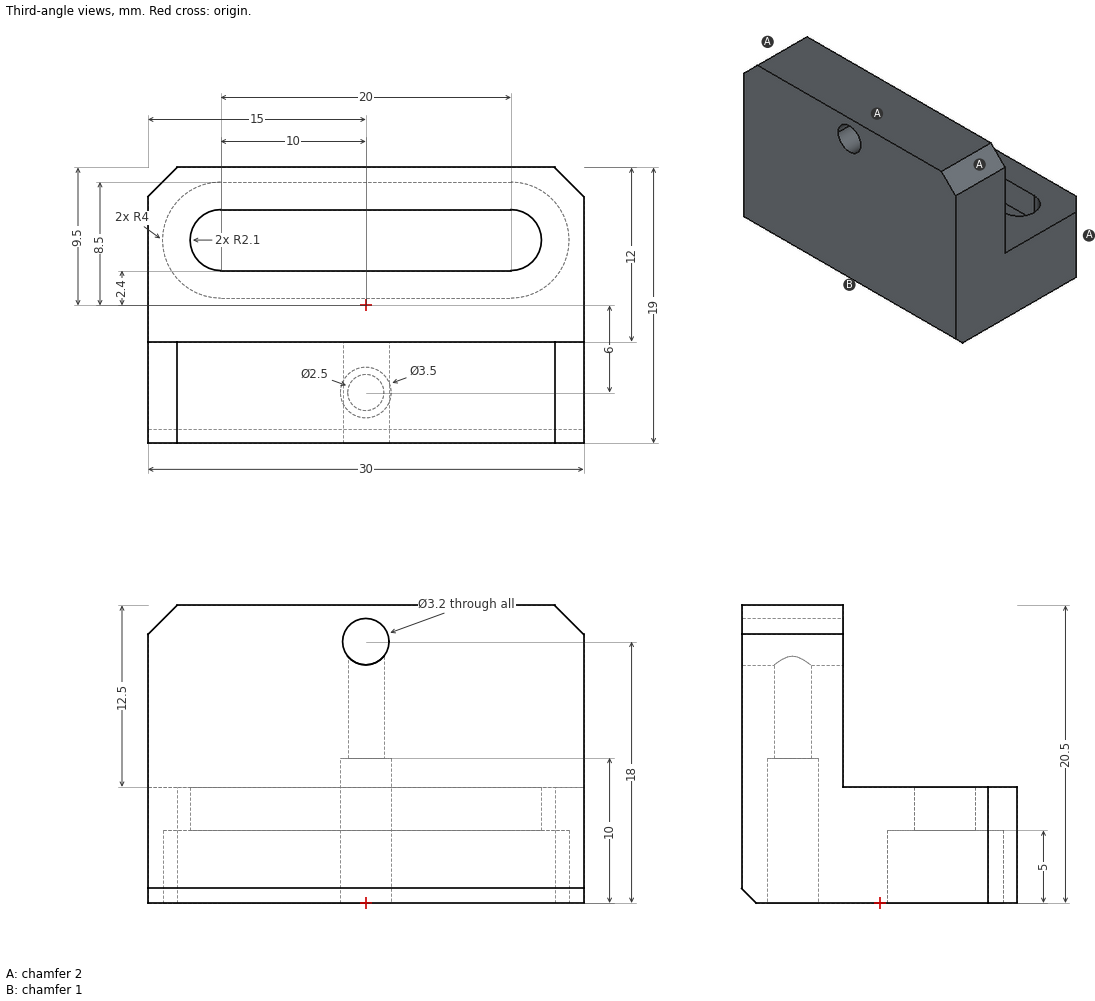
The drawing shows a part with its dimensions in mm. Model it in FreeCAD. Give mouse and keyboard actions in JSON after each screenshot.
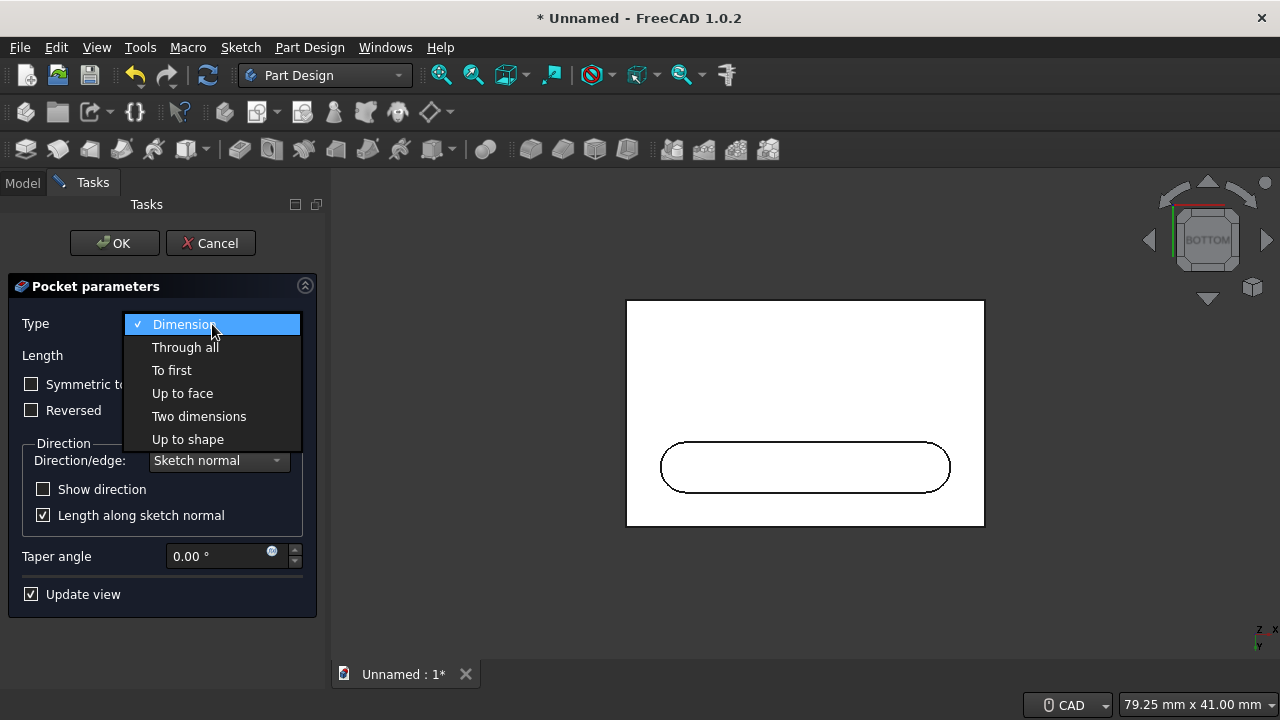
{"action": "left_click", "coordinate": [212, 348]}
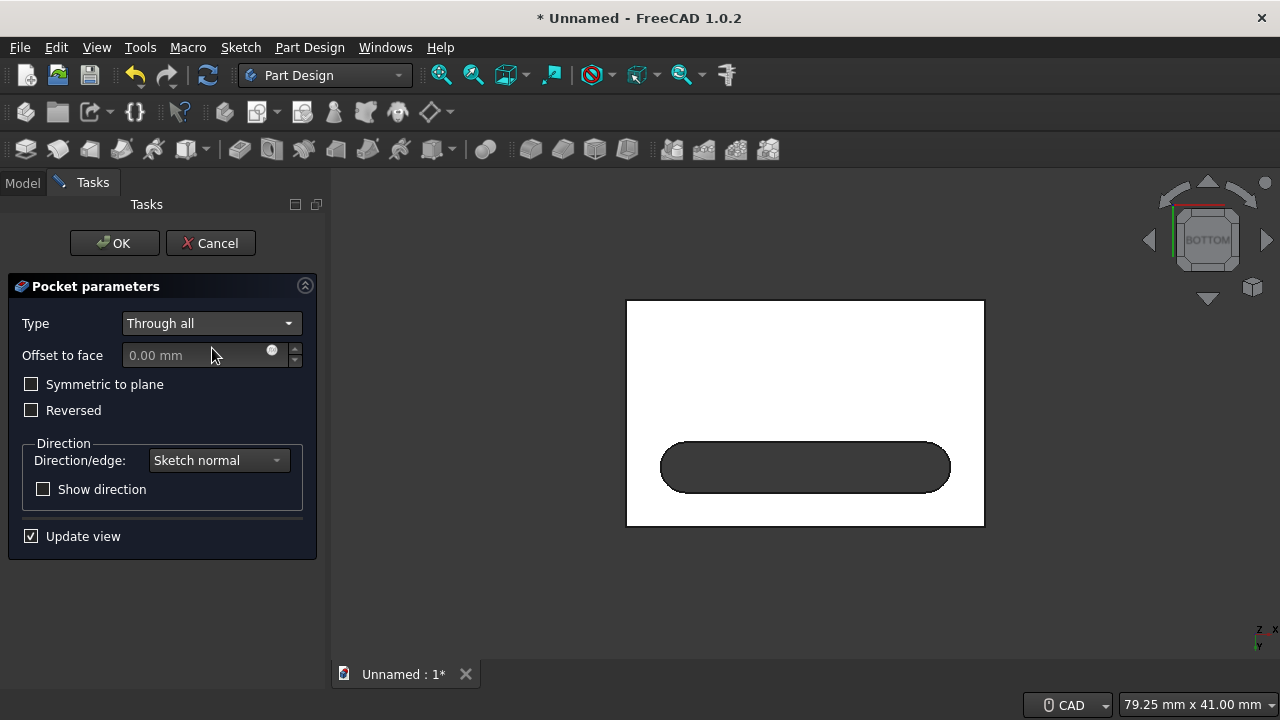
{"action": "left_click", "coordinate": [115, 243]}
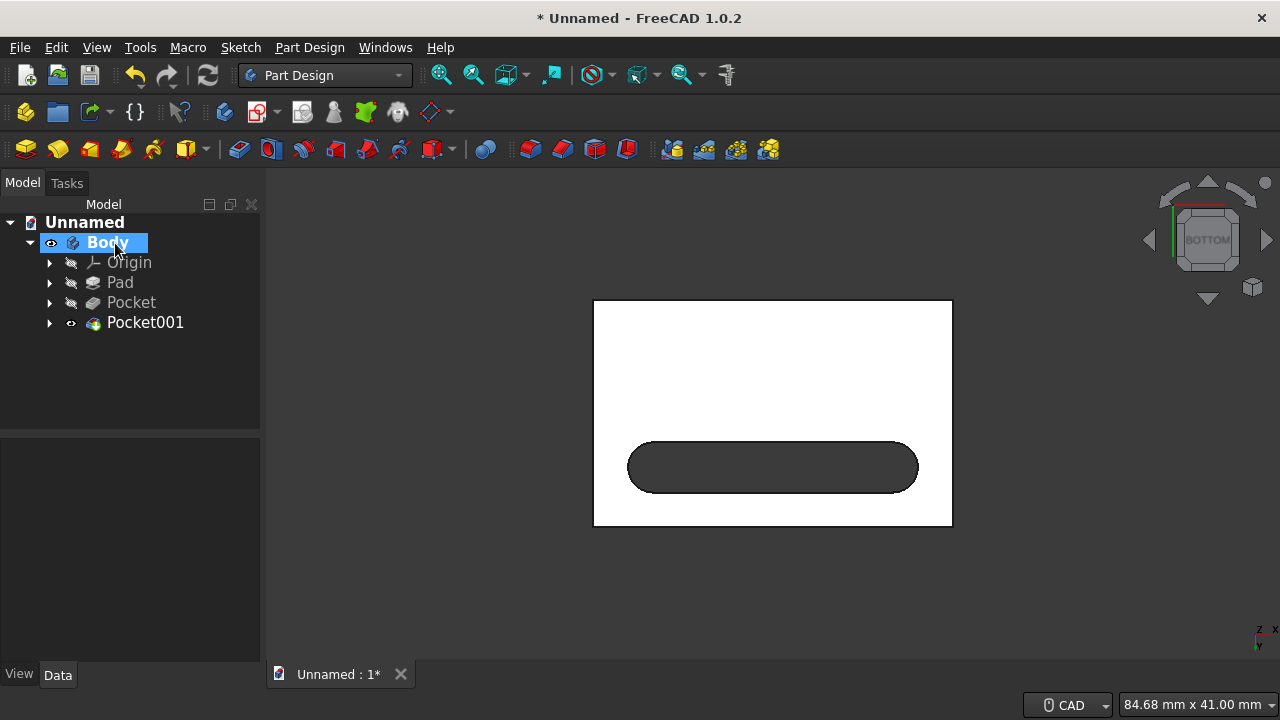
{"action": "left_click", "coordinate": [258, 112]}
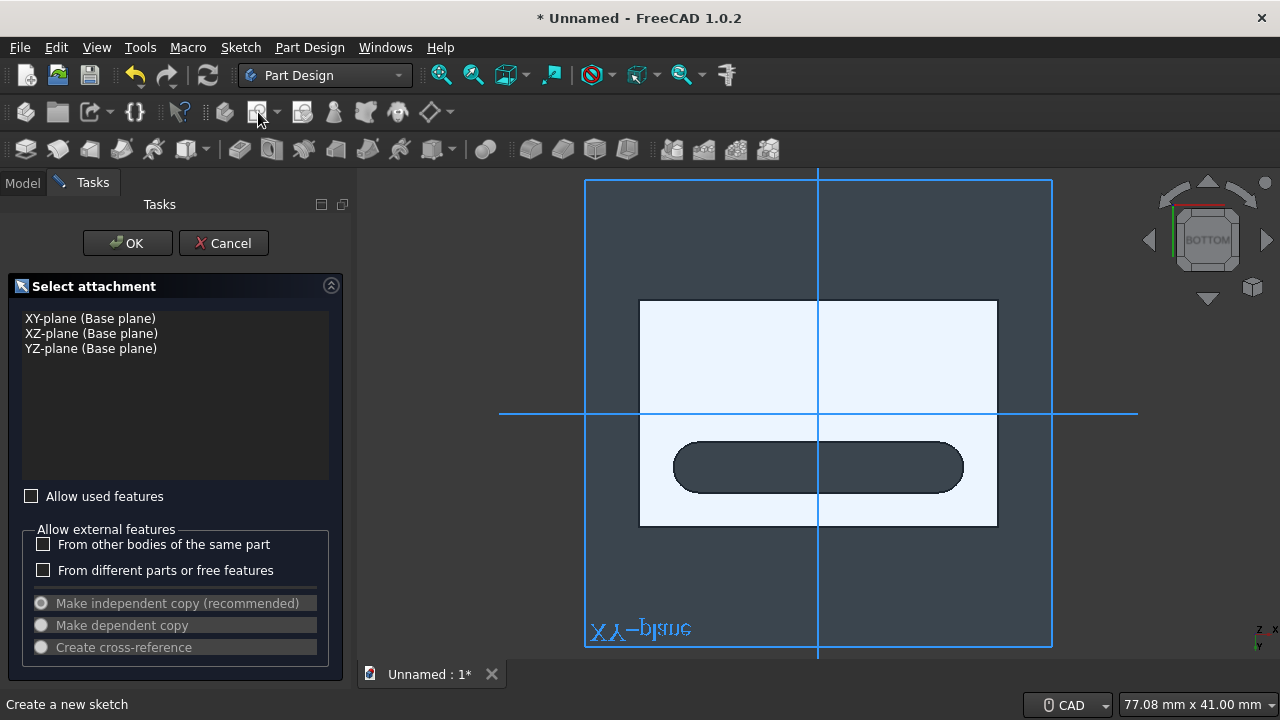
{"action": "left_click", "coordinate": [82, 318]}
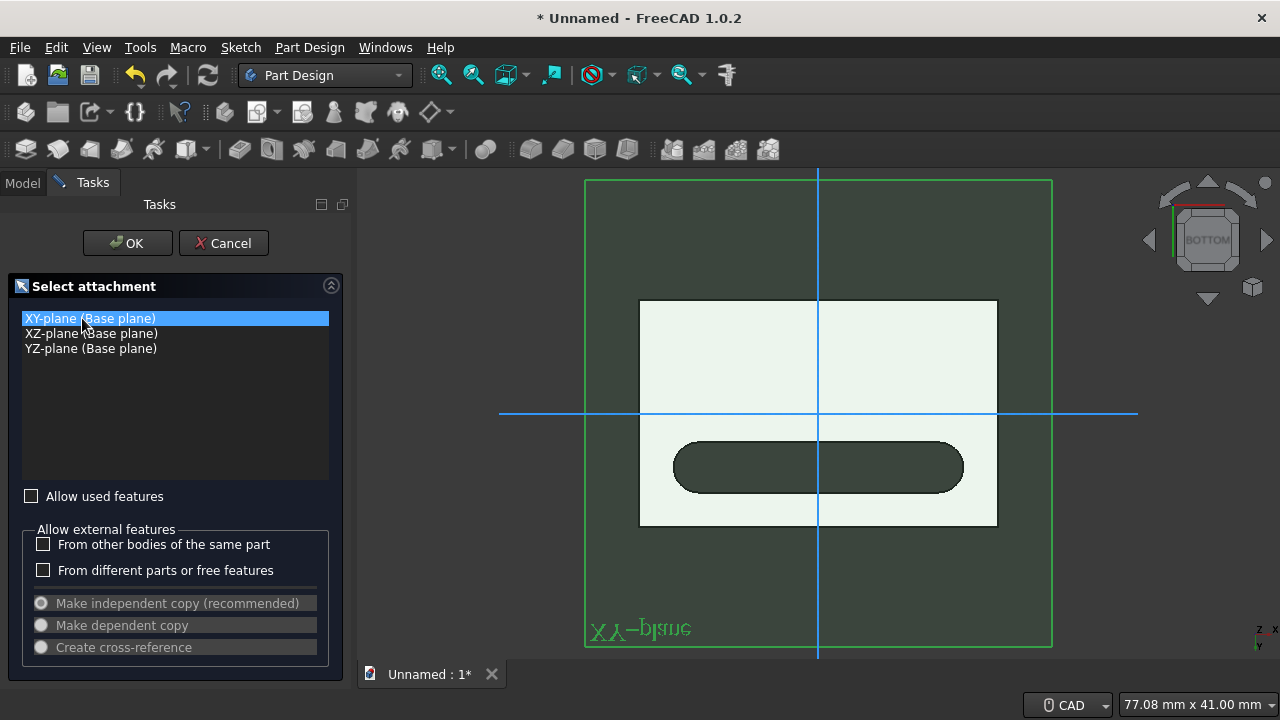
{"action": "left_click", "coordinate": [128, 243]}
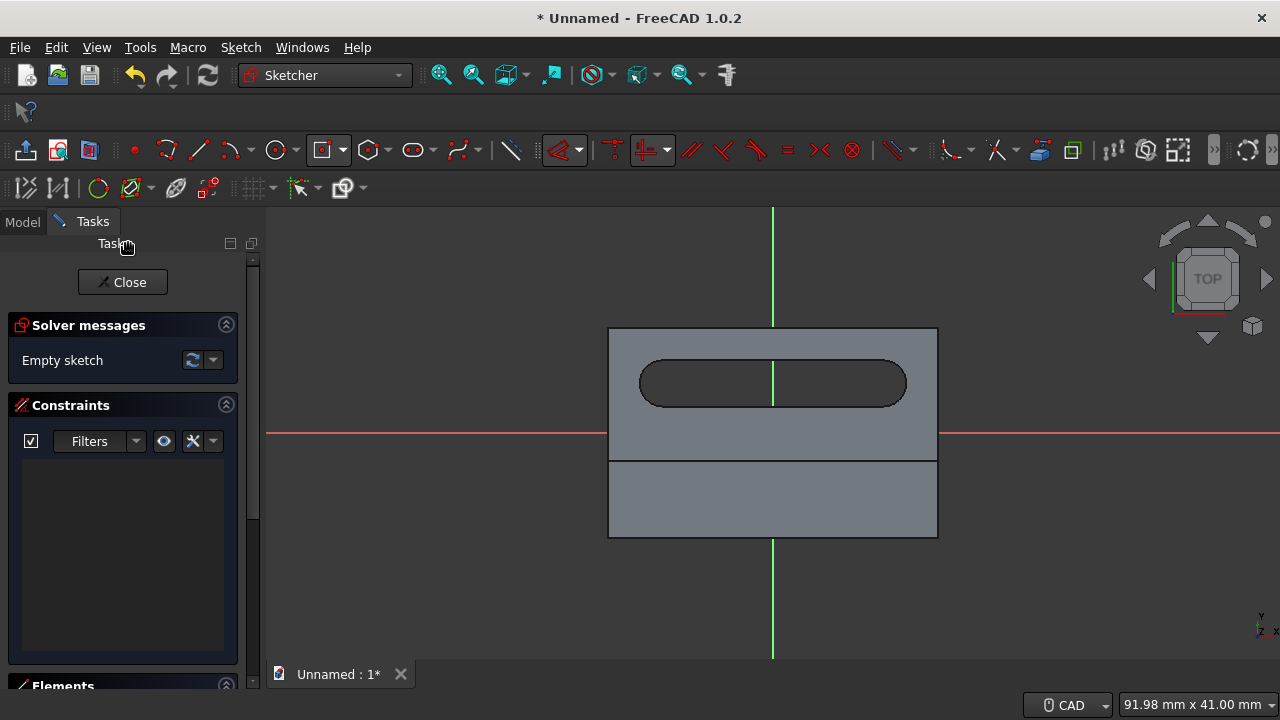
{"action": "left_click", "coordinate": [90, 150]}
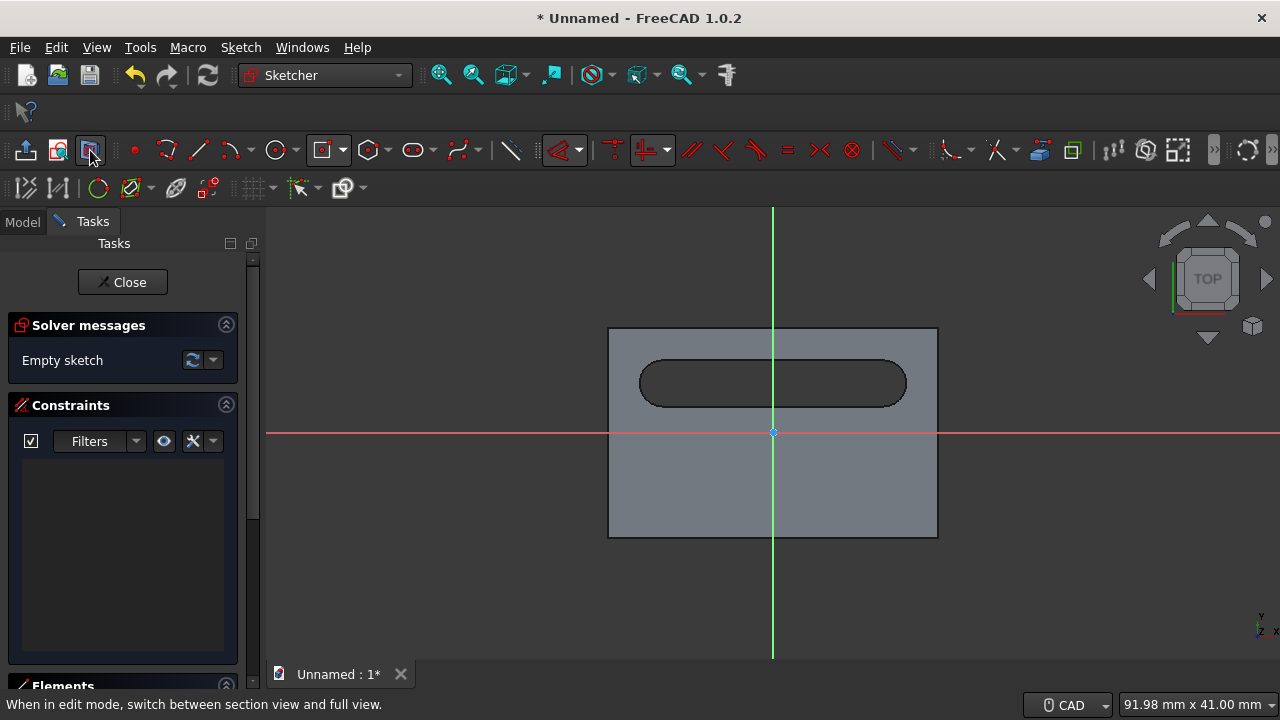
{"action": "scroll", "coordinate": [856, 329], "scroll_direction": "up", "scroll_amount": 3}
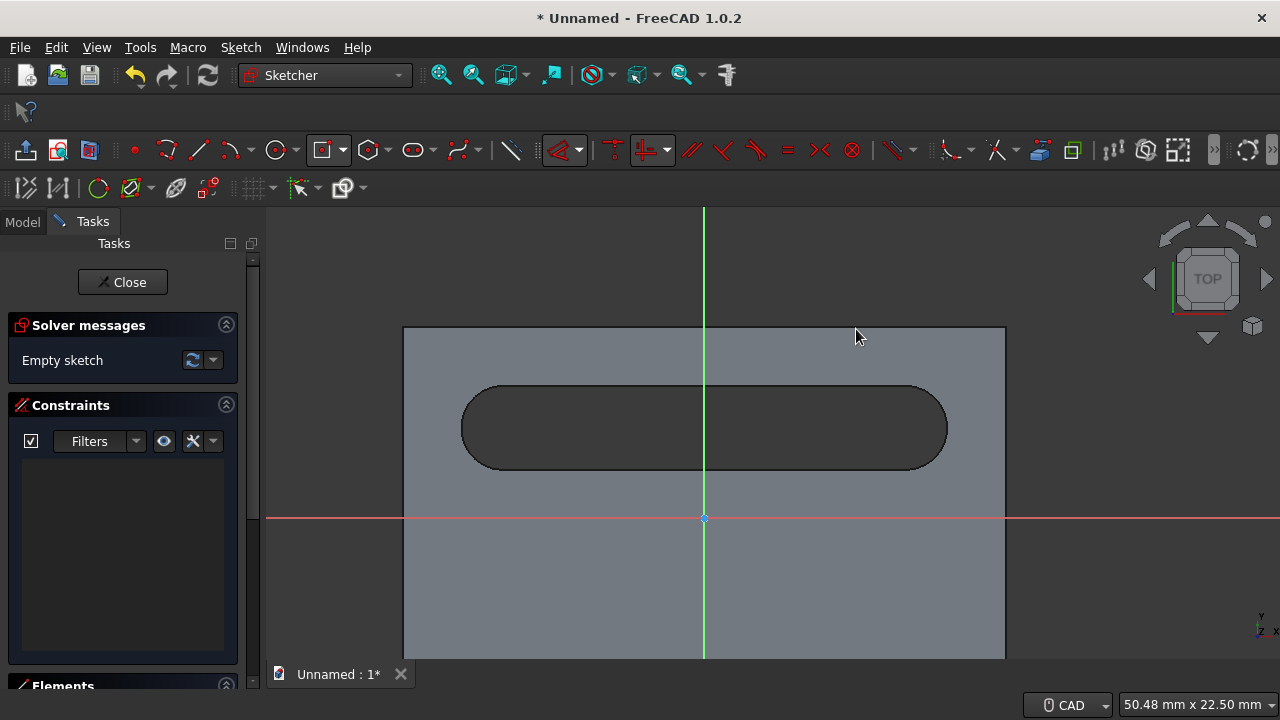
{"action": "left_click", "coordinate": [414, 150]}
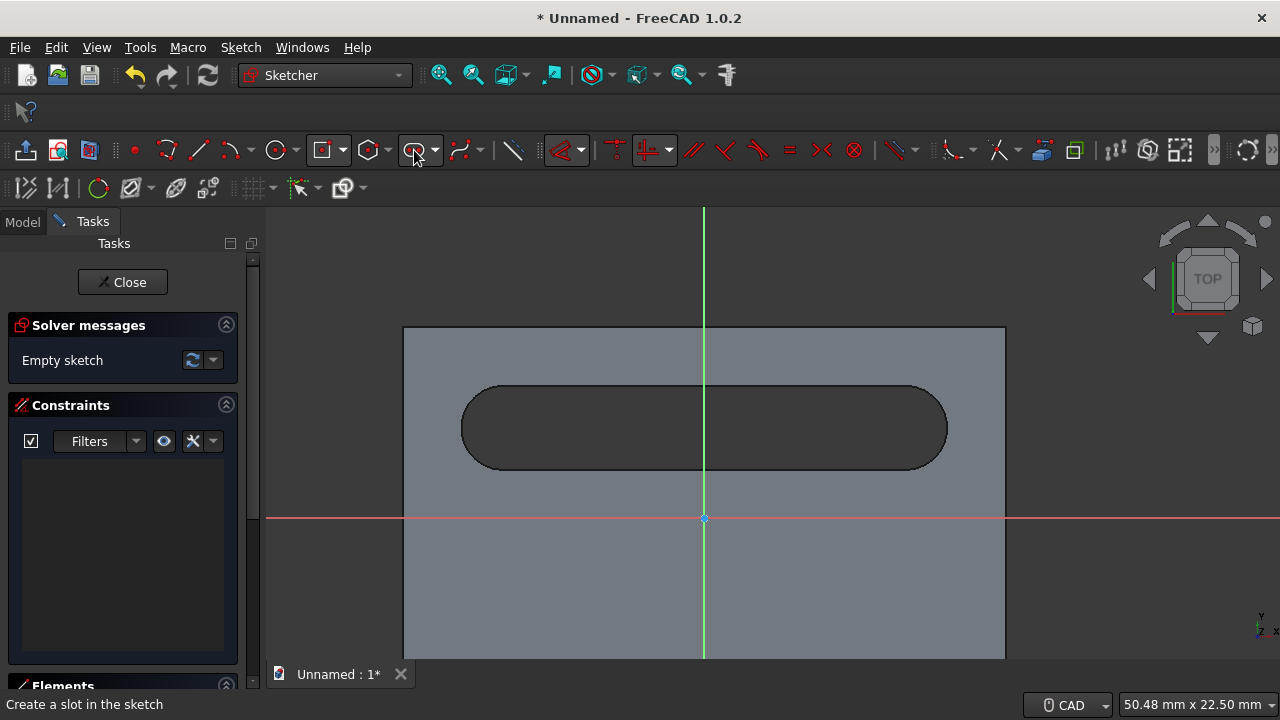
{"action": "left_click", "coordinate": [503, 428]}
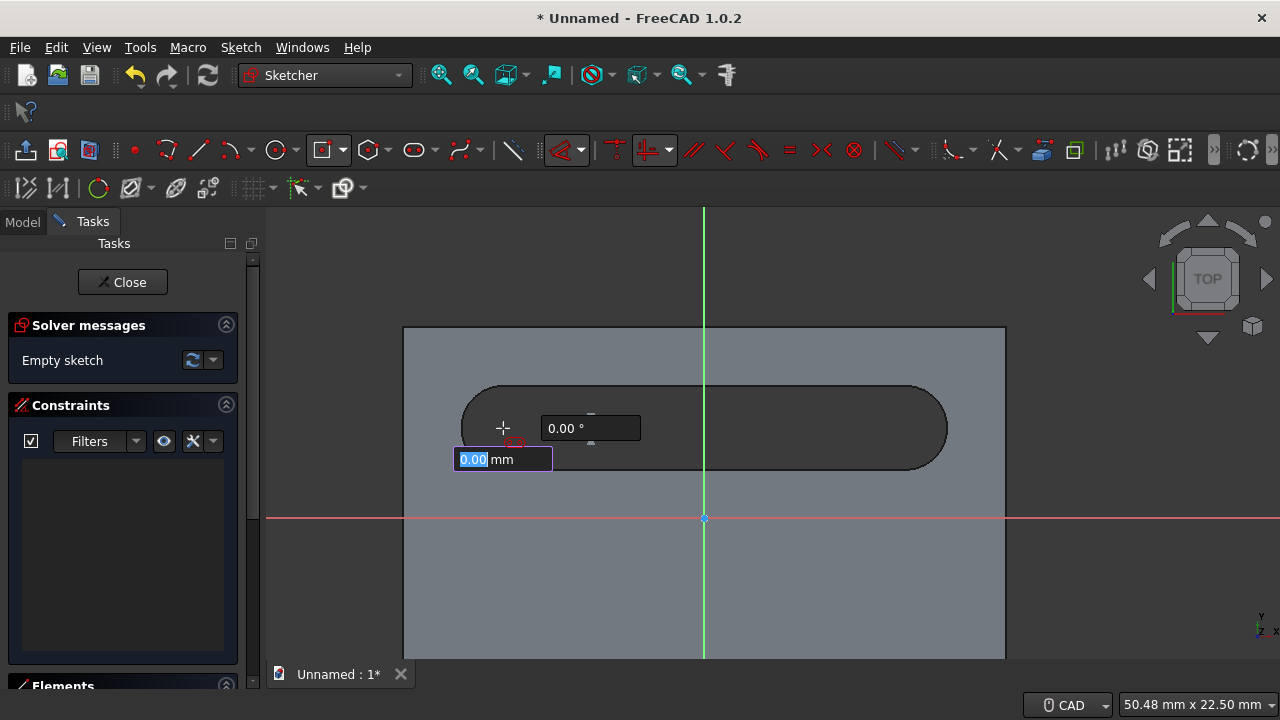
{"action": "left_click", "coordinate": [905, 428]}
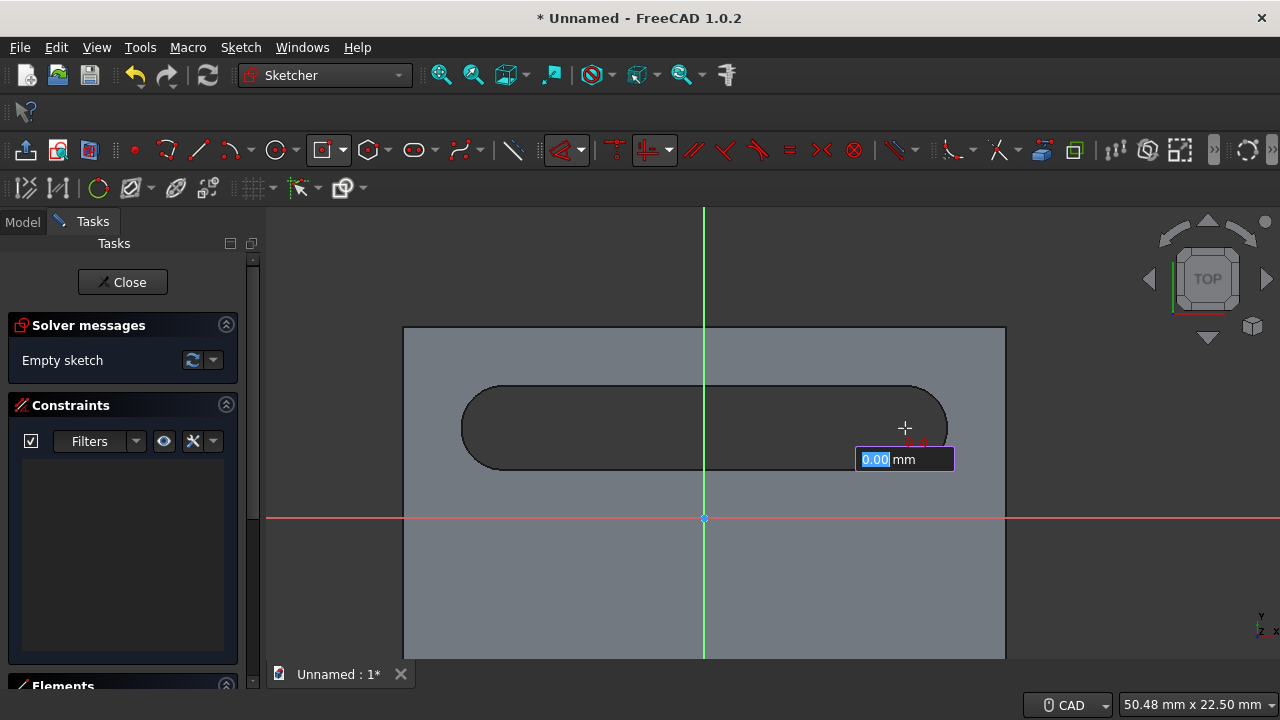
{"action": "left_click", "coordinate": [644, 348]}
{"action": "key", "text": "Escape"}